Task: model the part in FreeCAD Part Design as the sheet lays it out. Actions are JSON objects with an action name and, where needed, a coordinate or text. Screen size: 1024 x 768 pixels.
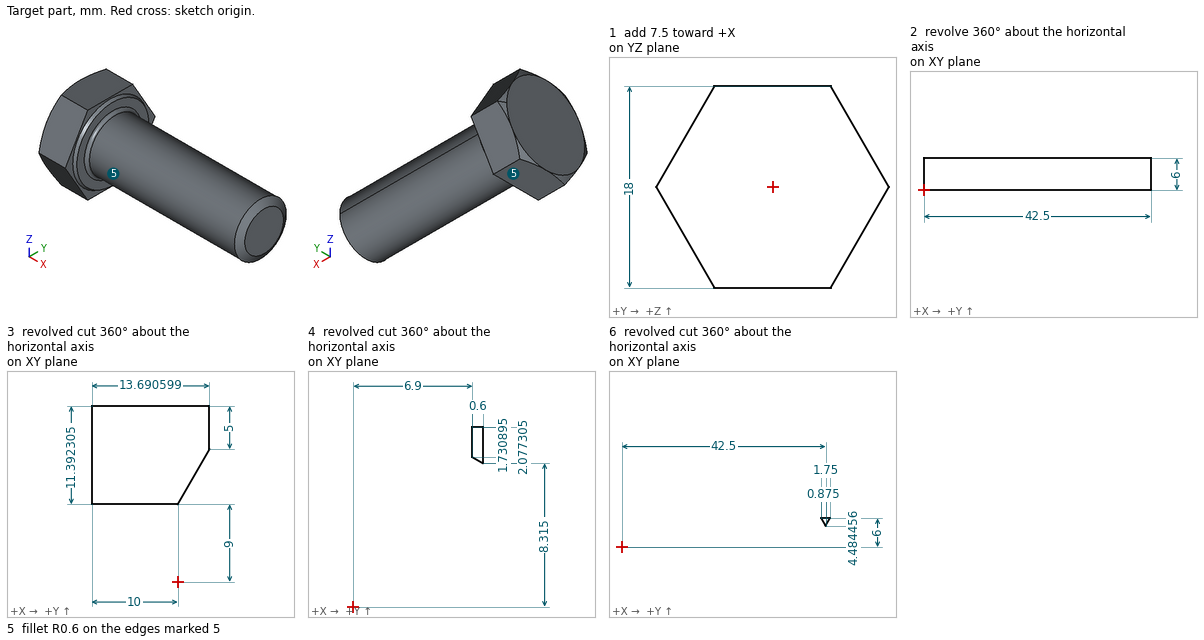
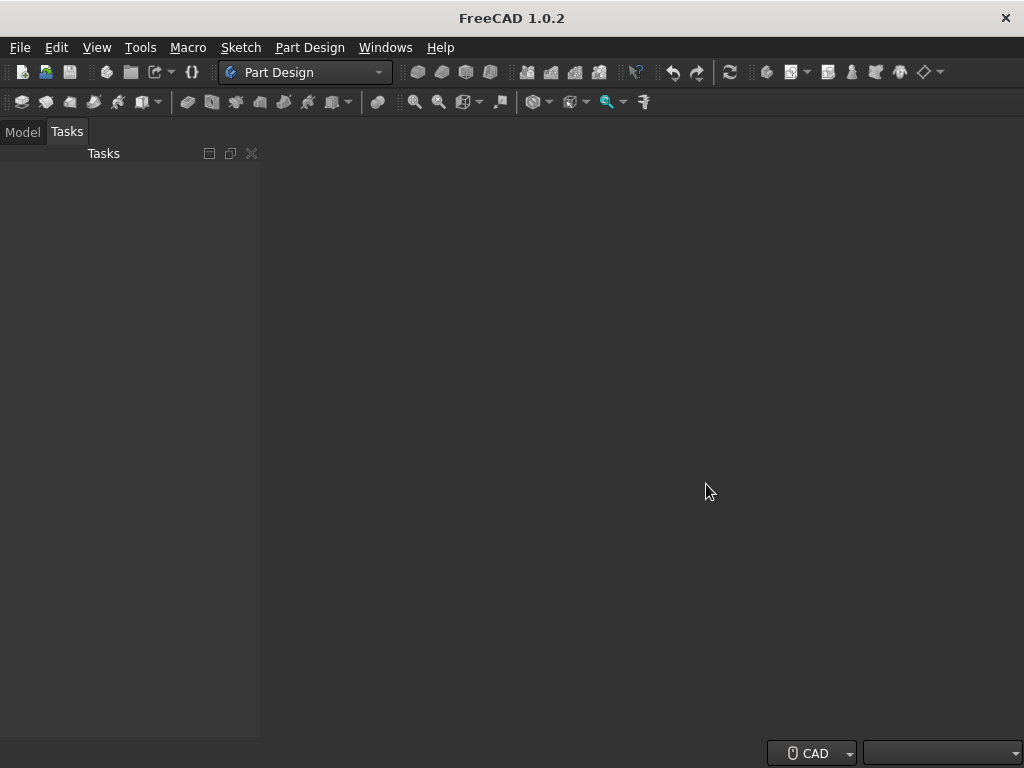
{"action": "left_click", "coordinate": [22, 72]}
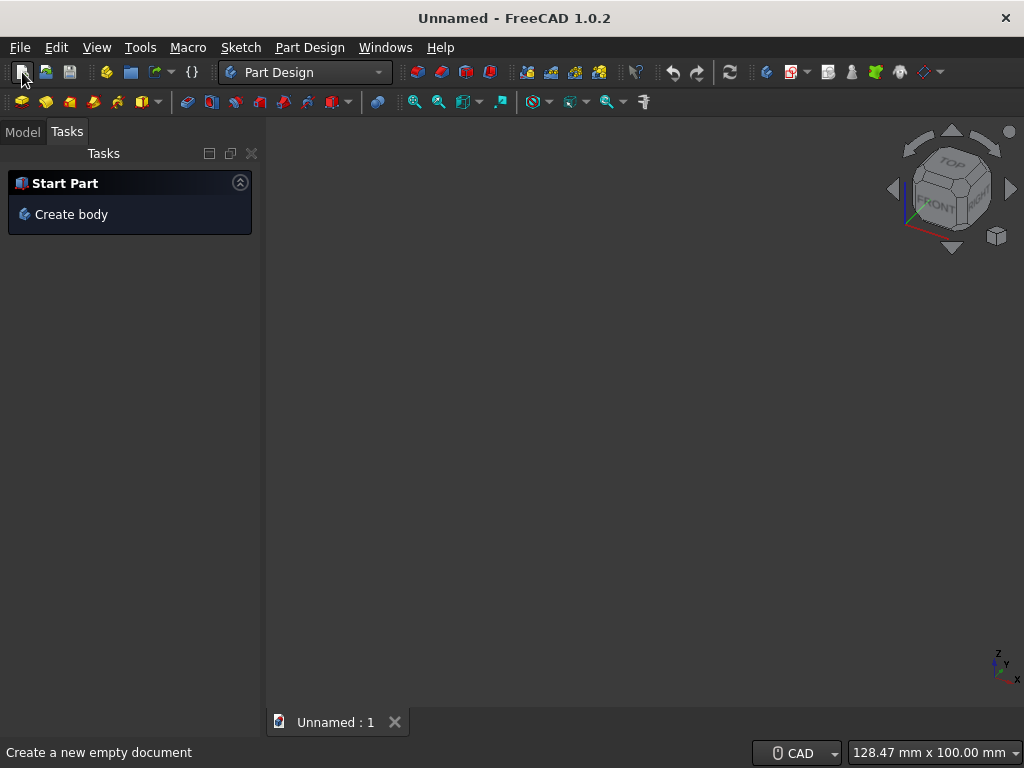
{"action": "left_click", "coordinate": [792, 72]}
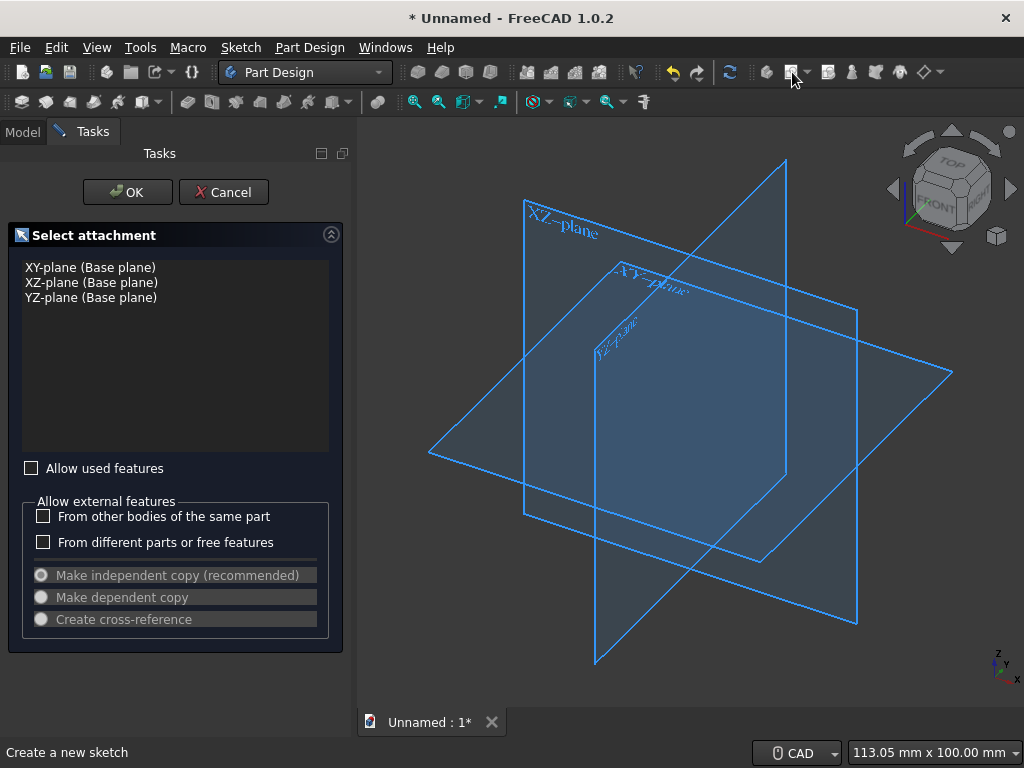
{"action": "left_click", "coordinate": [82, 298]}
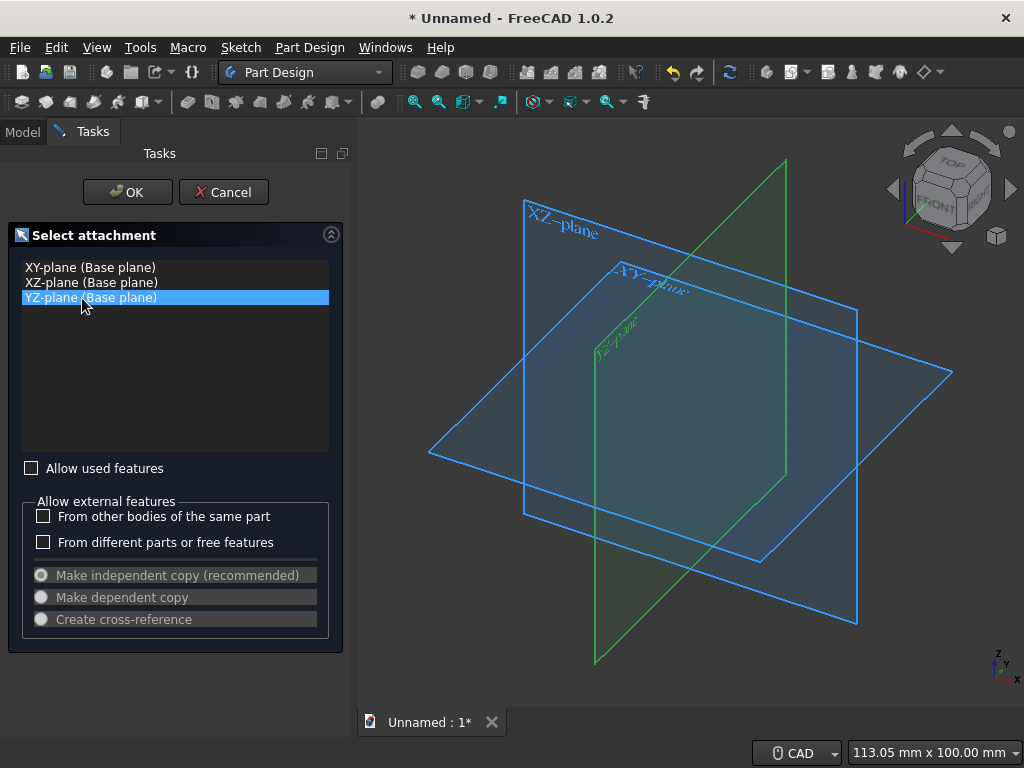
{"action": "left_click", "coordinate": [128, 192]}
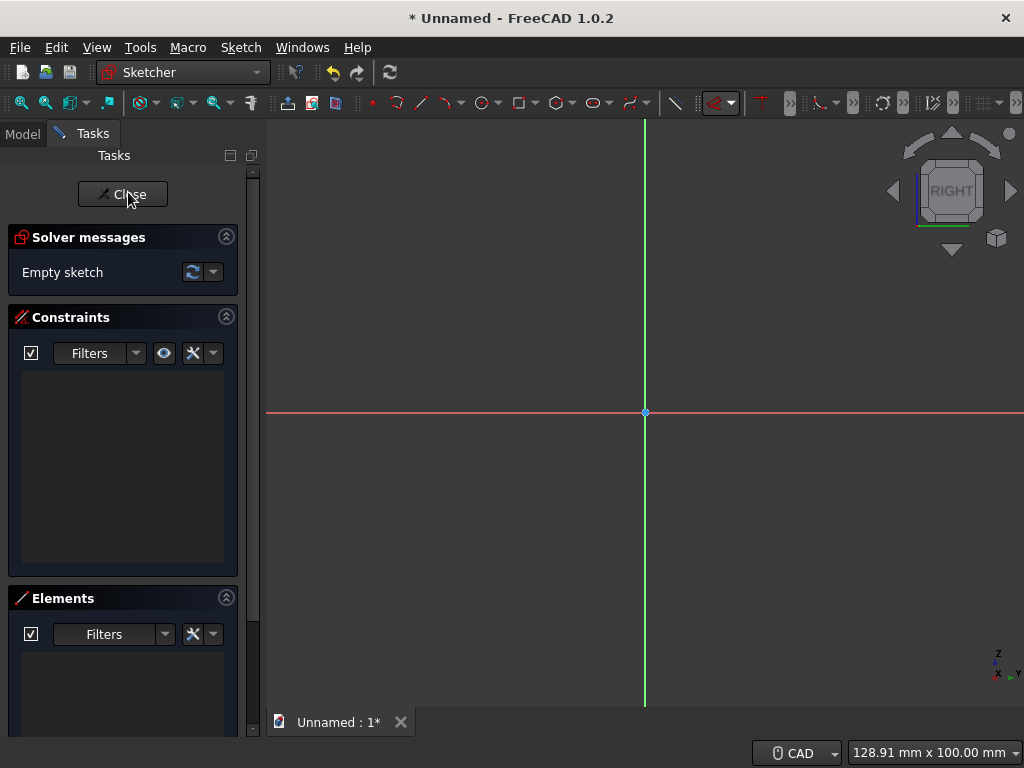
{"action": "scroll", "coordinate": [675, 413], "scroll_direction": "up", "scroll_amount": 6}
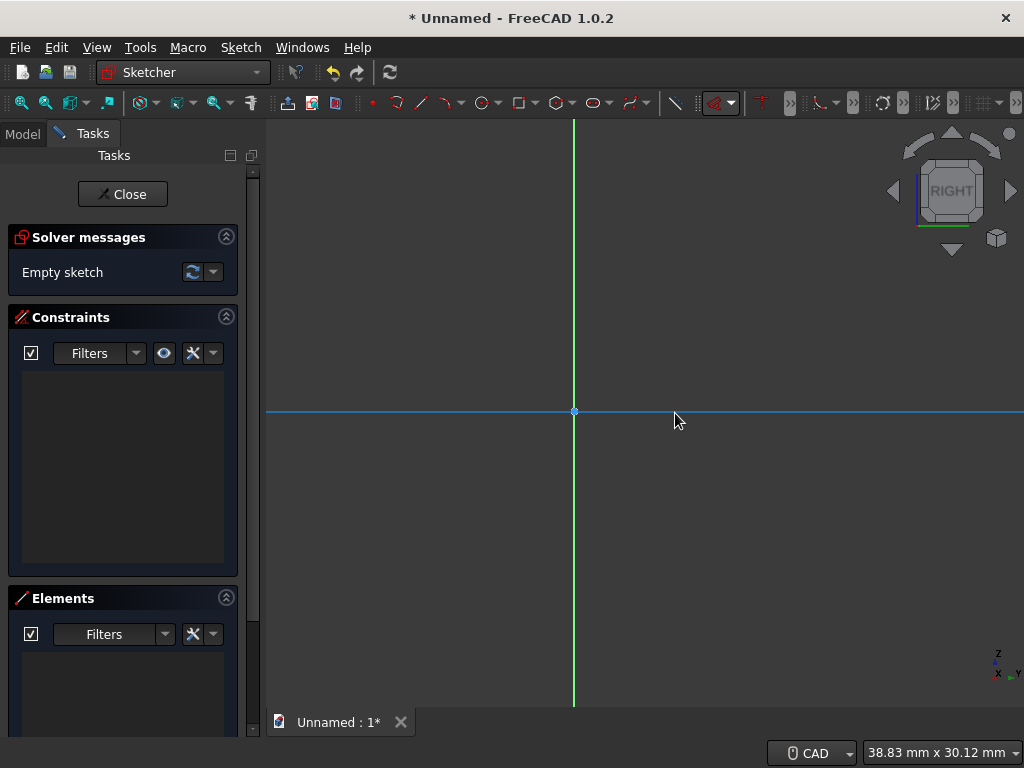
{"action": "left_click", "coordinate": [556, 104]}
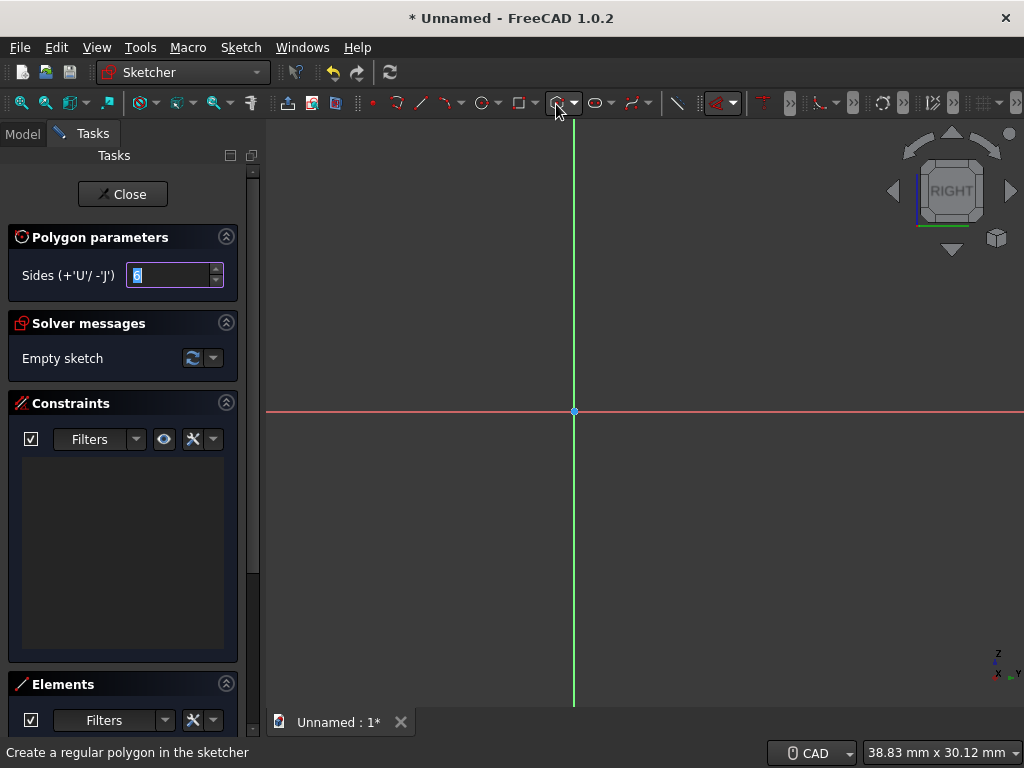
{"action": "left_click", "coordinate": [574, 412]}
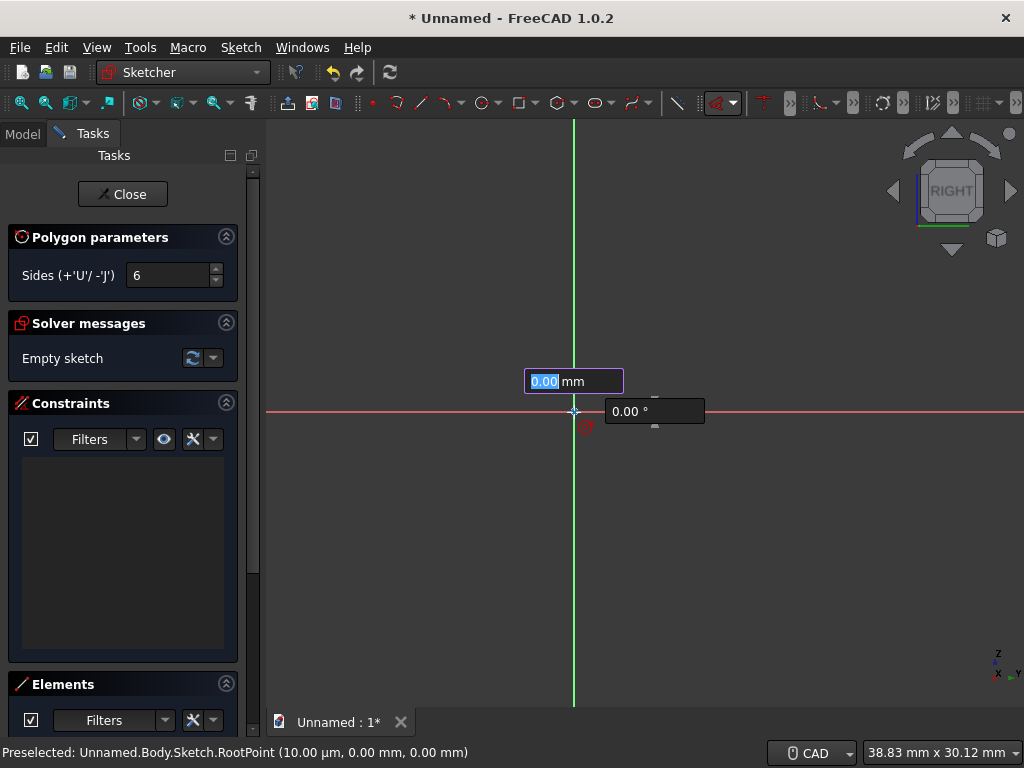
{"action": "left_click", "coordinate": [777, 412]}
{"action": "right_click", "coordinate": [777, 412]}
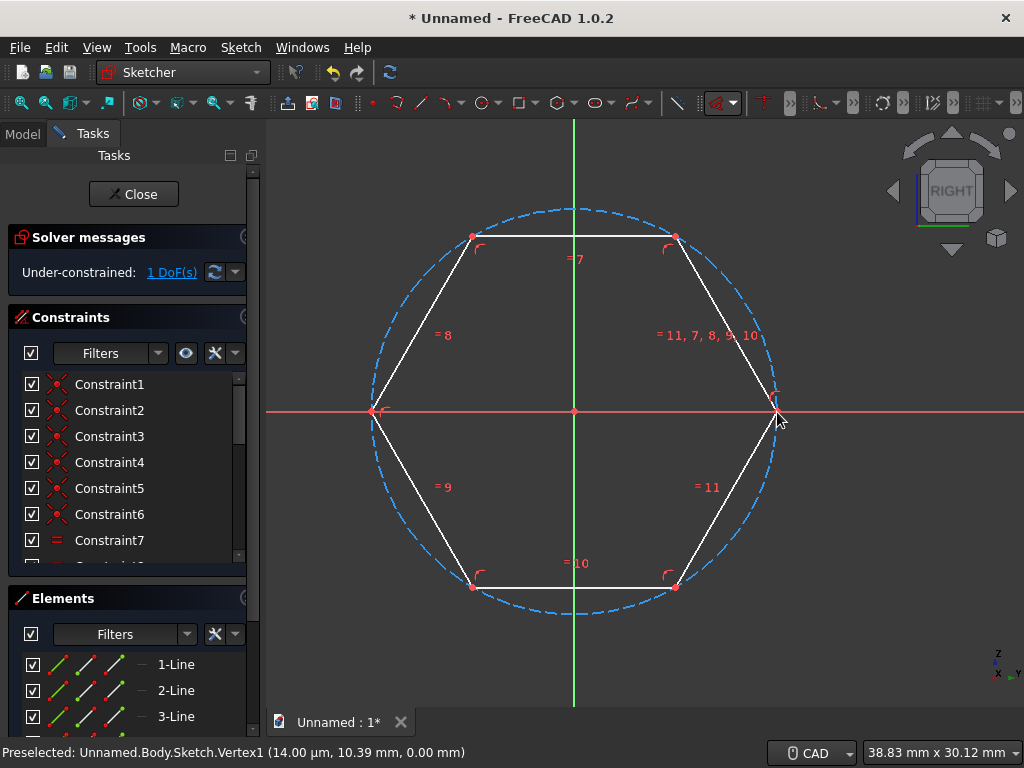
{"action": "left_click", "coordinate": [716, 104]}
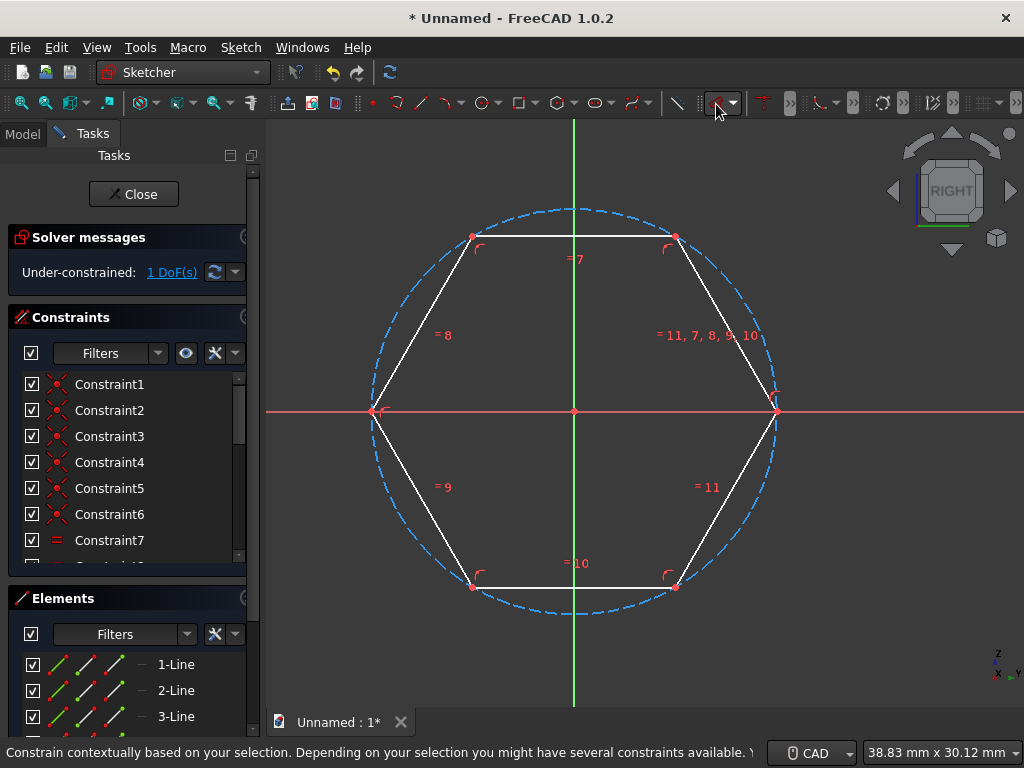
{"action": "left_click", "coordinate": [473, 588]}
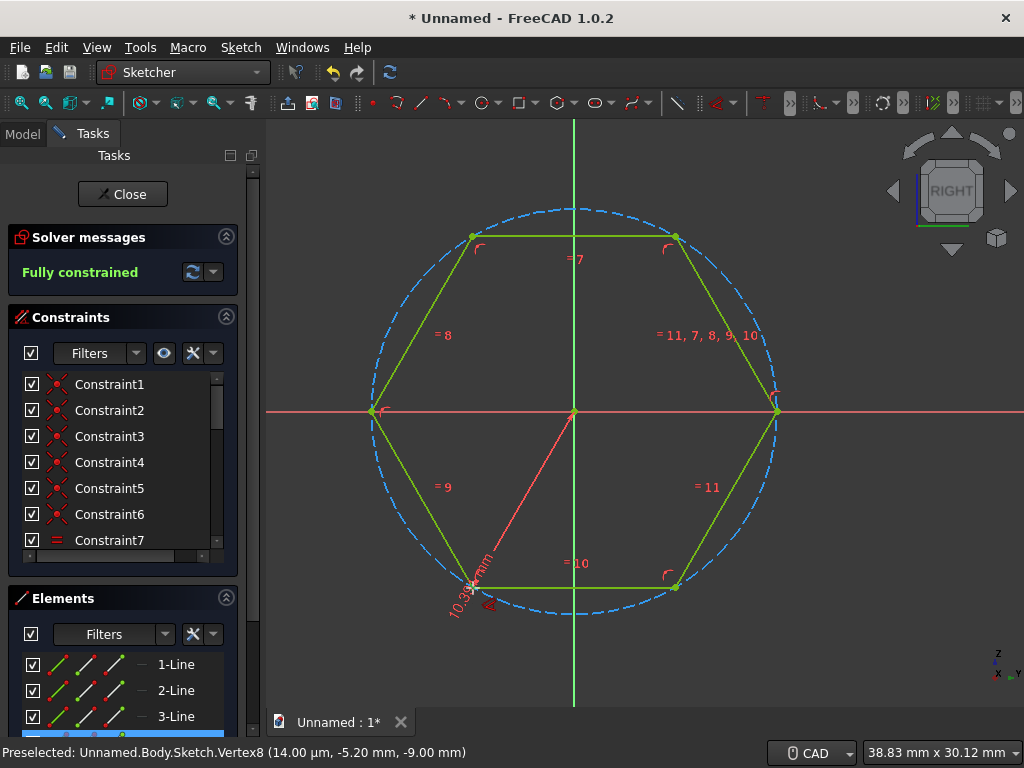
{"action": "left_click", "coordinate": [676, 236]}
{"action": "left_click", "coordinate": [710, 331]}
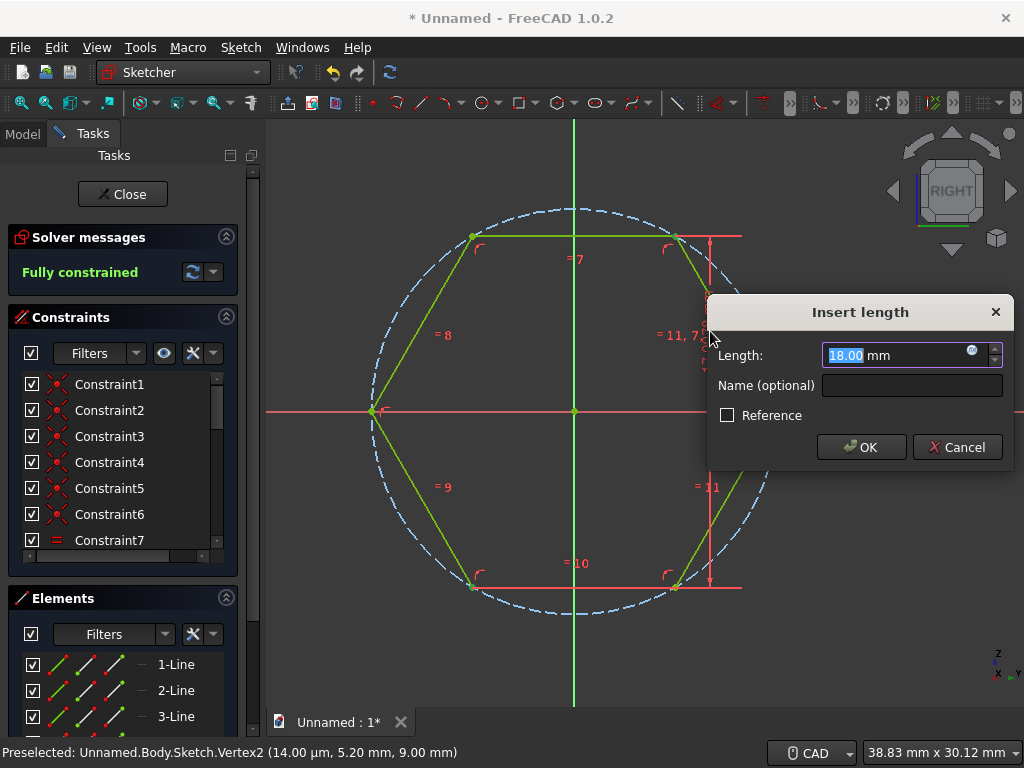
{"action": "type", "text": "18"}
{"action": "key", "text": "Return"}
{"action": "key", "text": "Escape"}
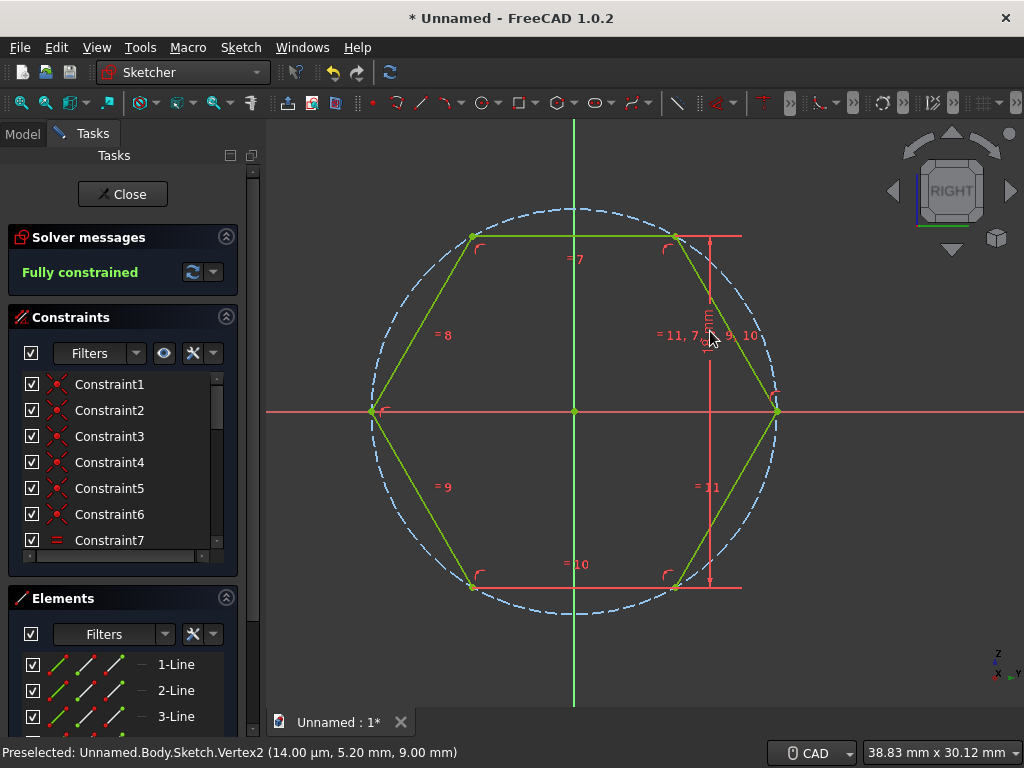
{"action": "left_click", "coordinate": [123, 194]}